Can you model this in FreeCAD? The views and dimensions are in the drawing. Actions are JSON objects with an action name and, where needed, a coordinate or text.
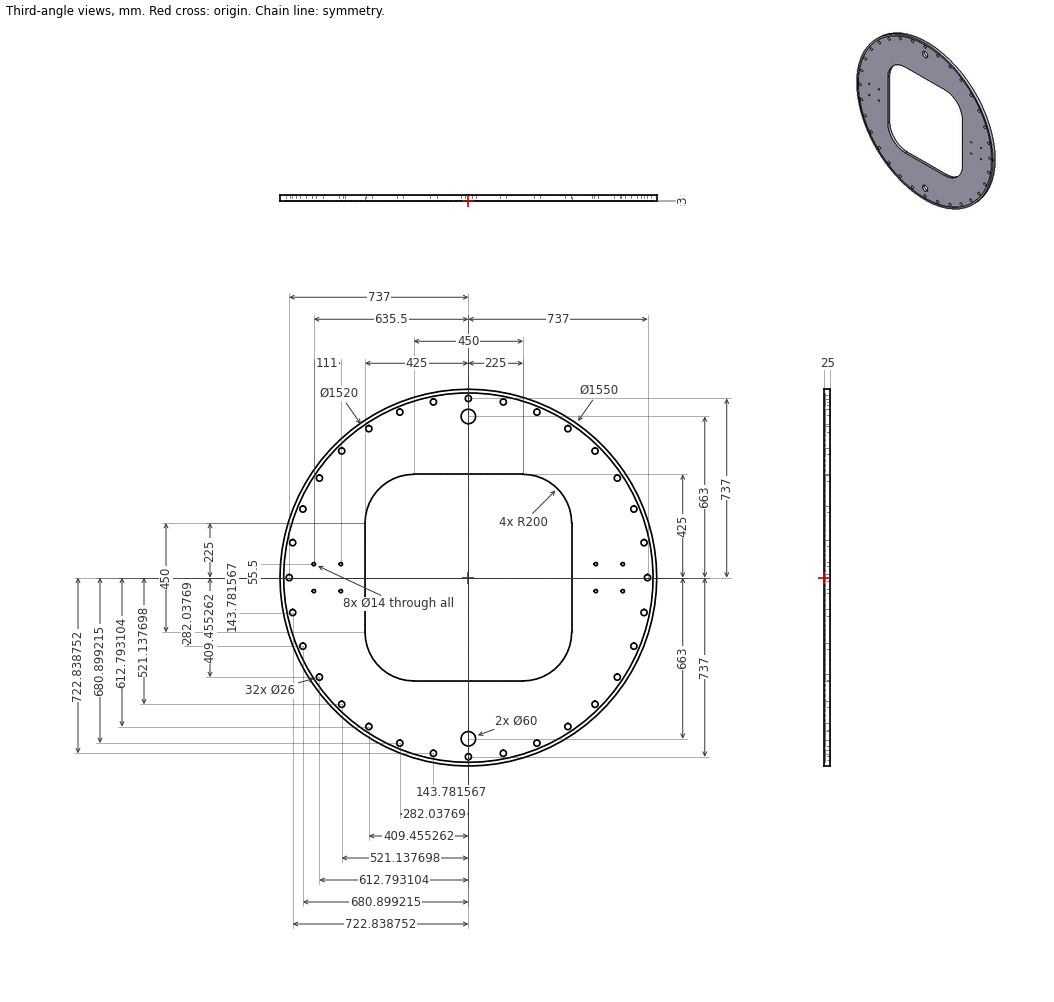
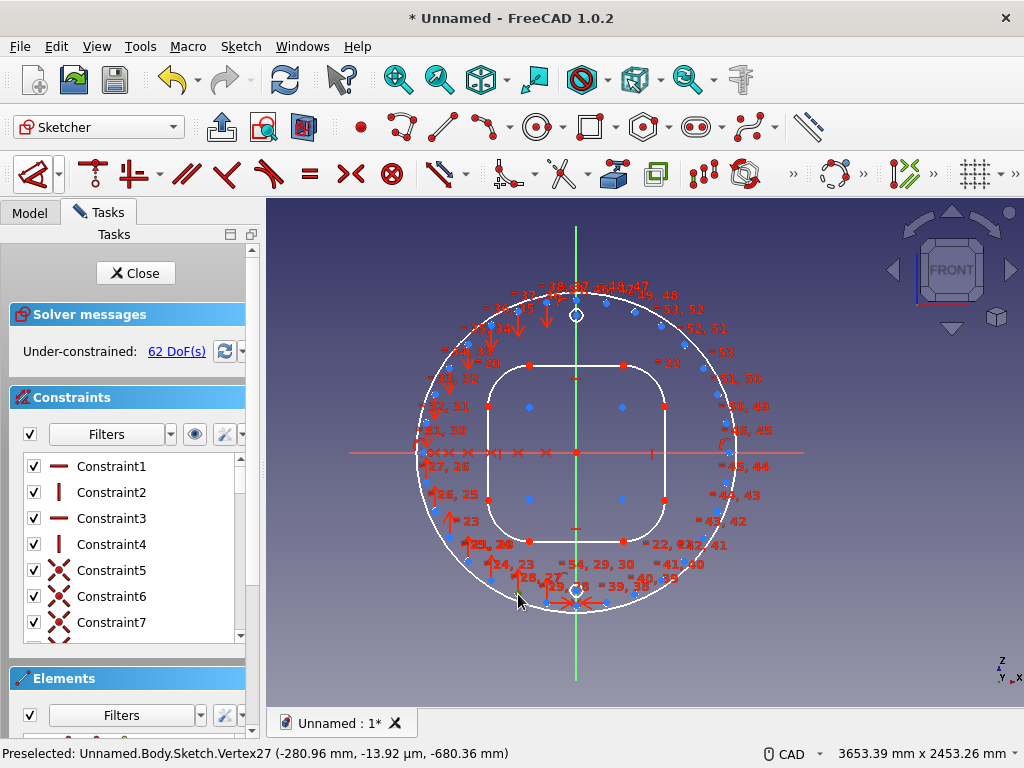
{"action": "left_click", "coordinate": [635, 595]}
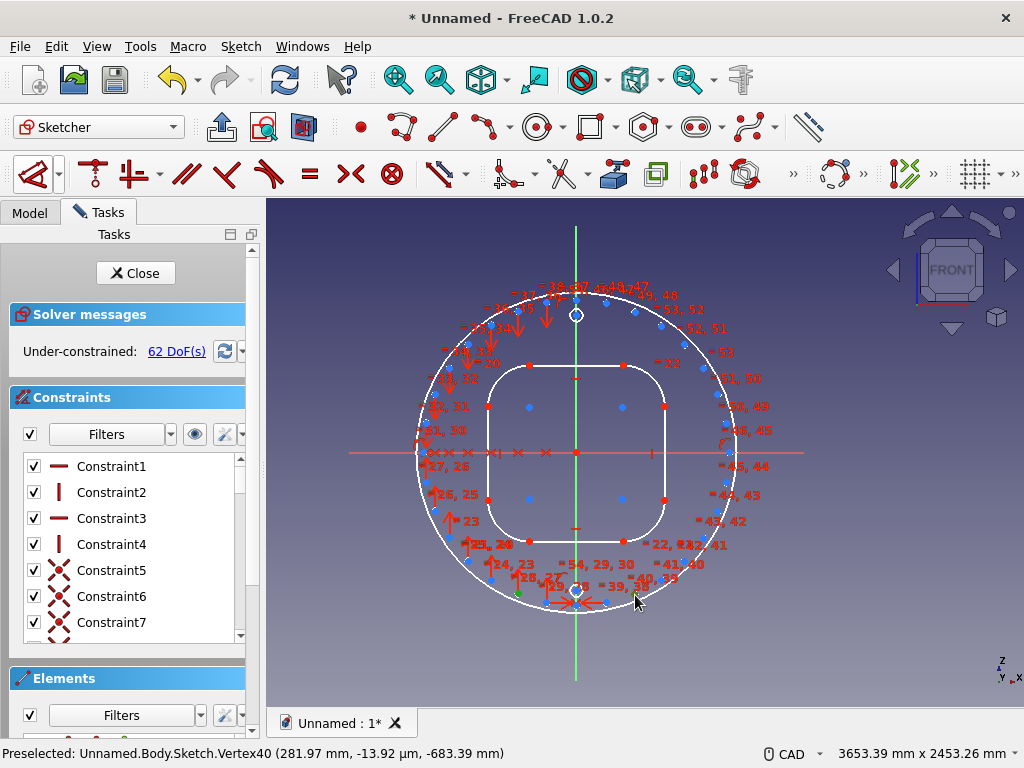
{"action": "left_click", "coordinate": [576, 647]}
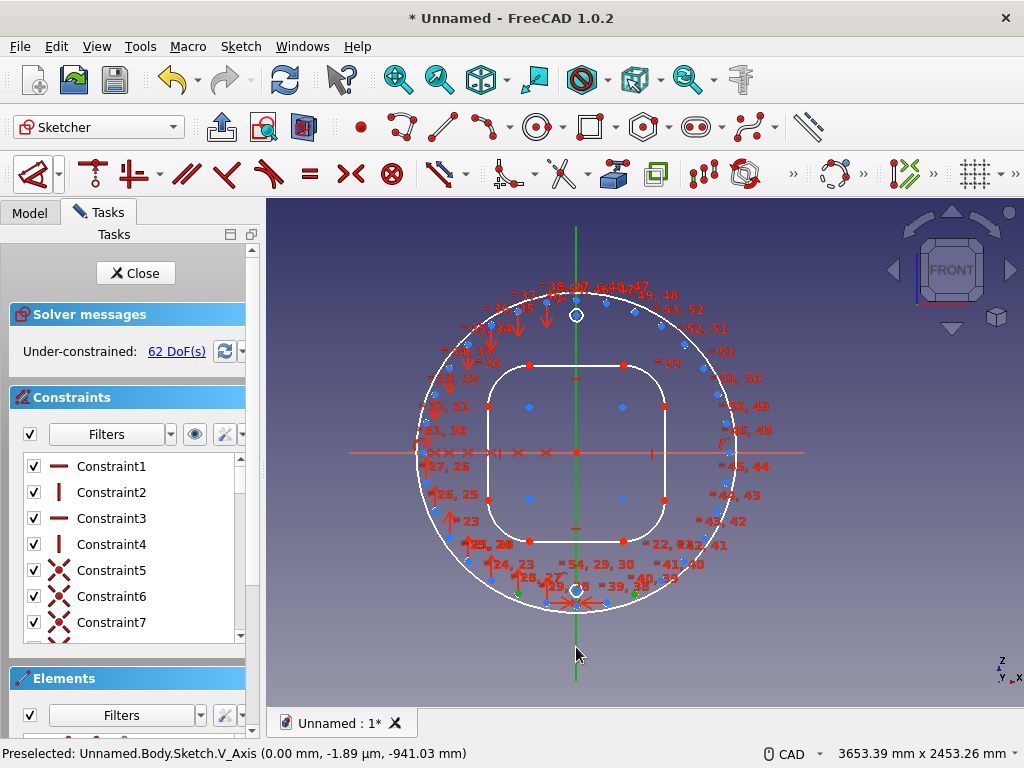
{"action": "left_click", "coordinate": [351, 174]}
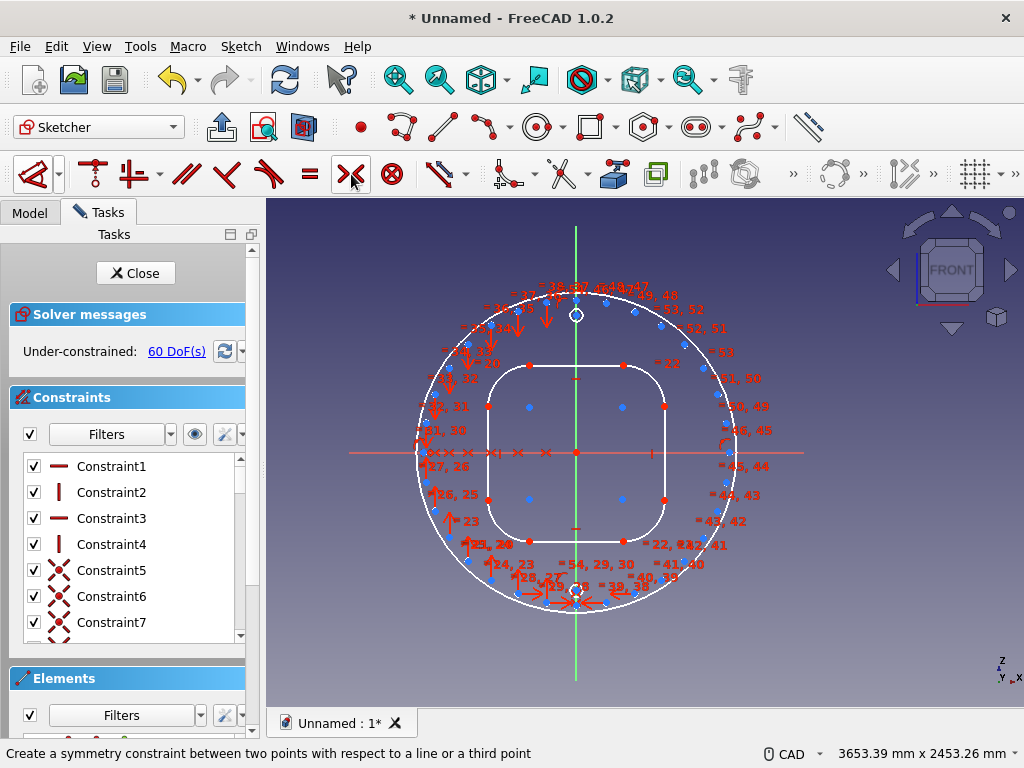
{"action": "left_click", "coordinate": [491, 580]}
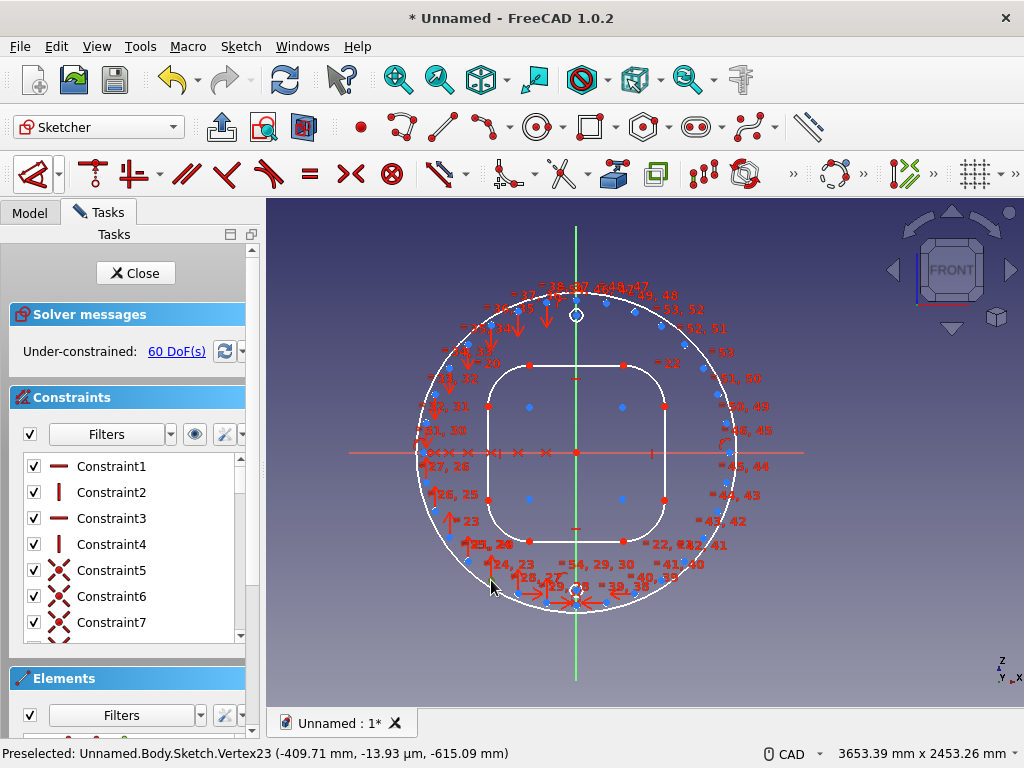
{"action": "left_click", "coordinate": [662, 580]}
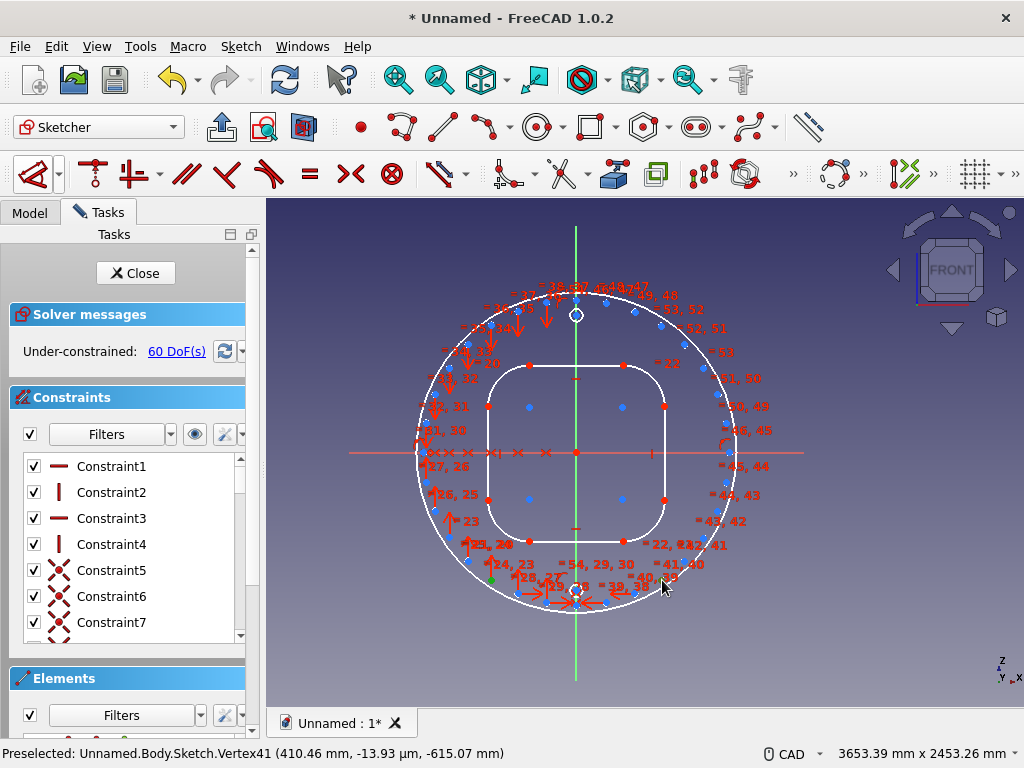
{"action": "left_click", "coordinate": [576, 647]}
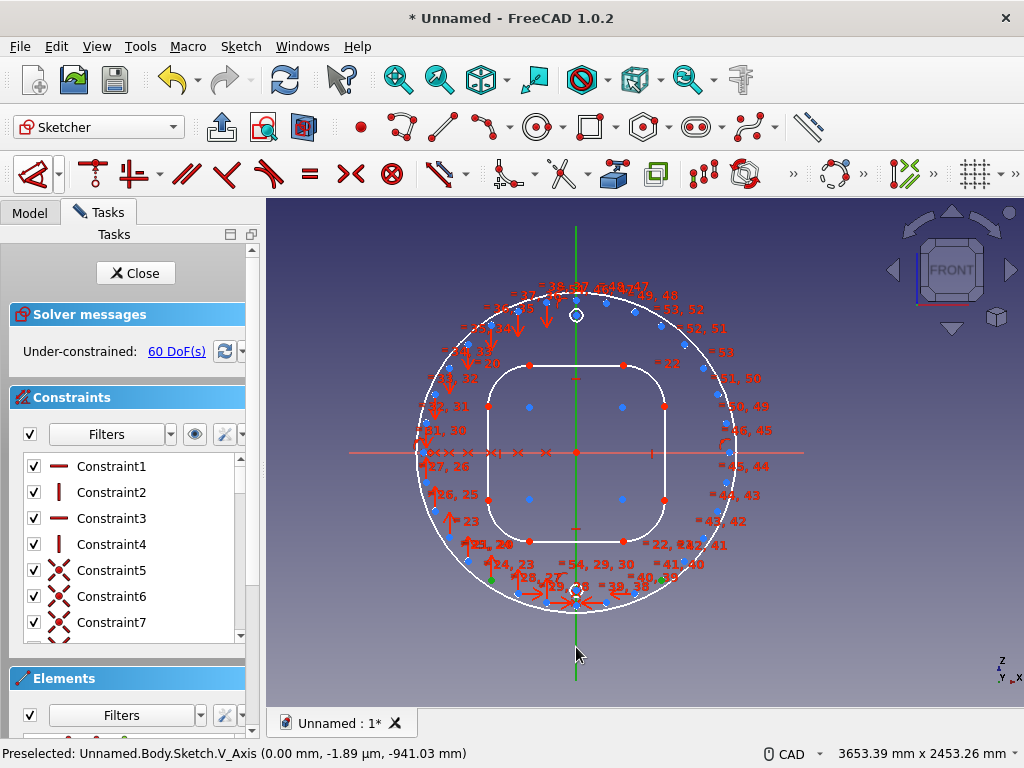
{"action": "left_click", "coordinate": [351, 174]}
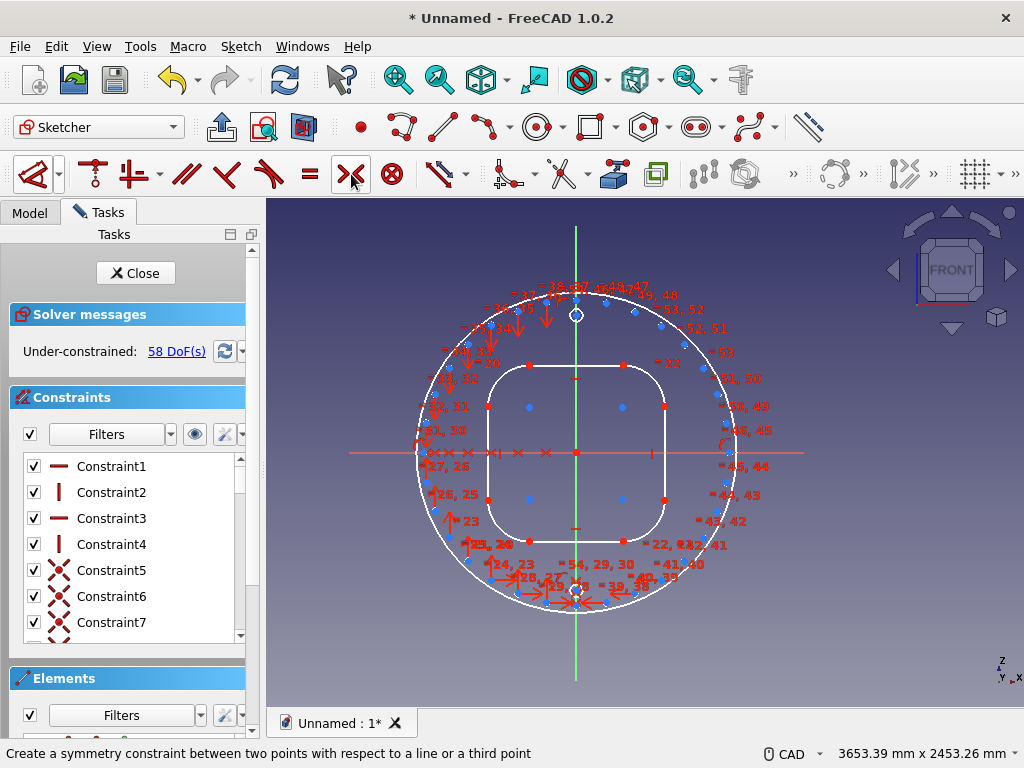
{"action": "left_click", "coordinate": [468, 561]}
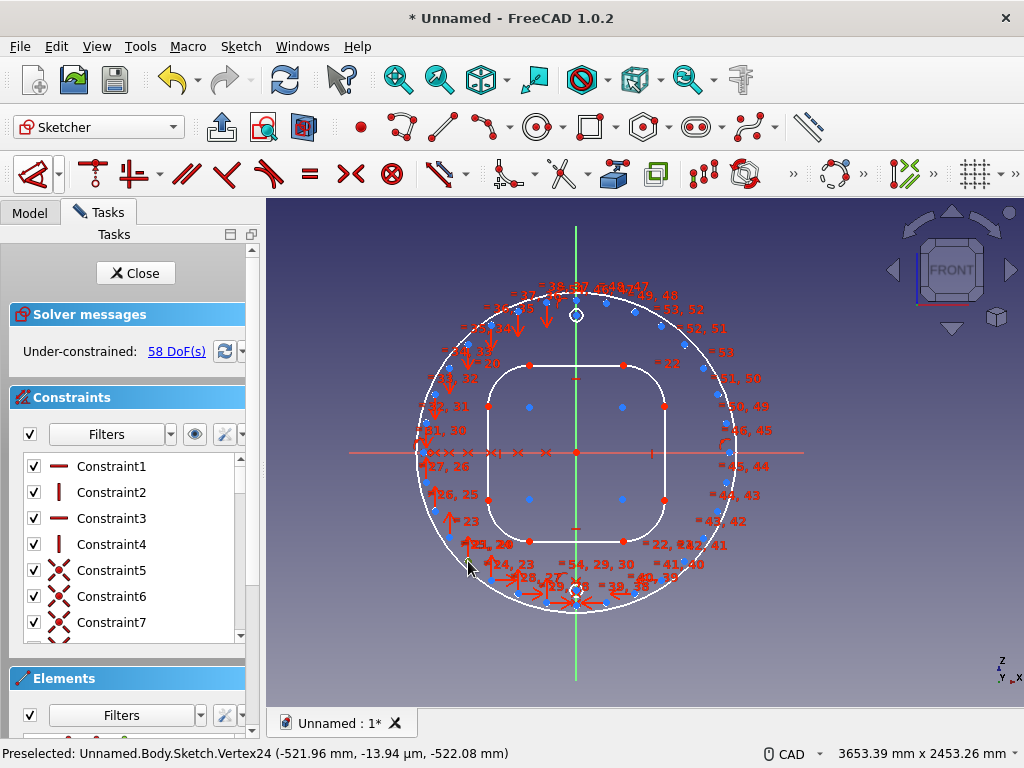
{"action": "left_click", "coordinate": [684, 561]}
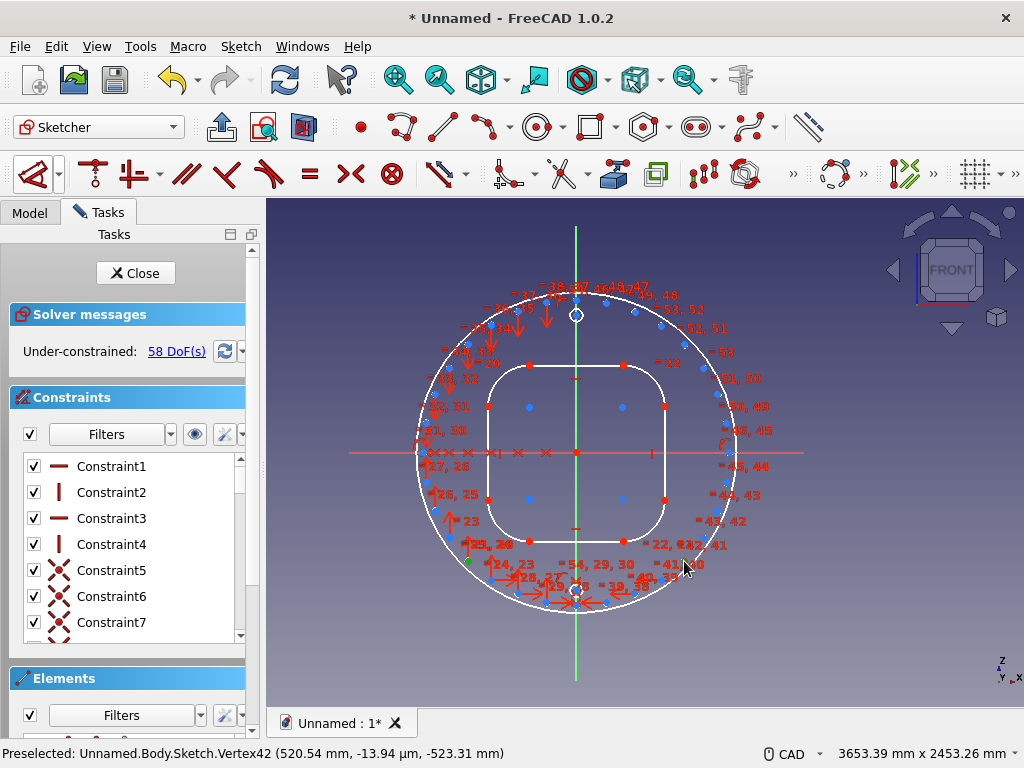
{"action": "left_click", "coordinate": [576, 647]}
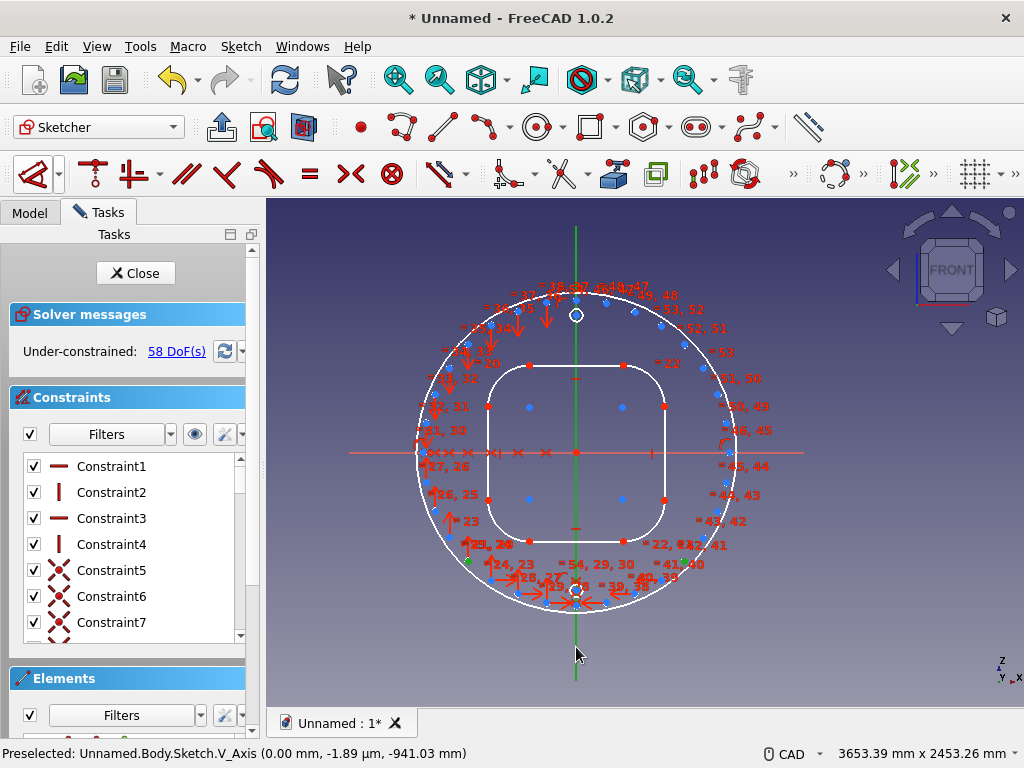
{"action": "left_click", "coordinate": [351, 174]}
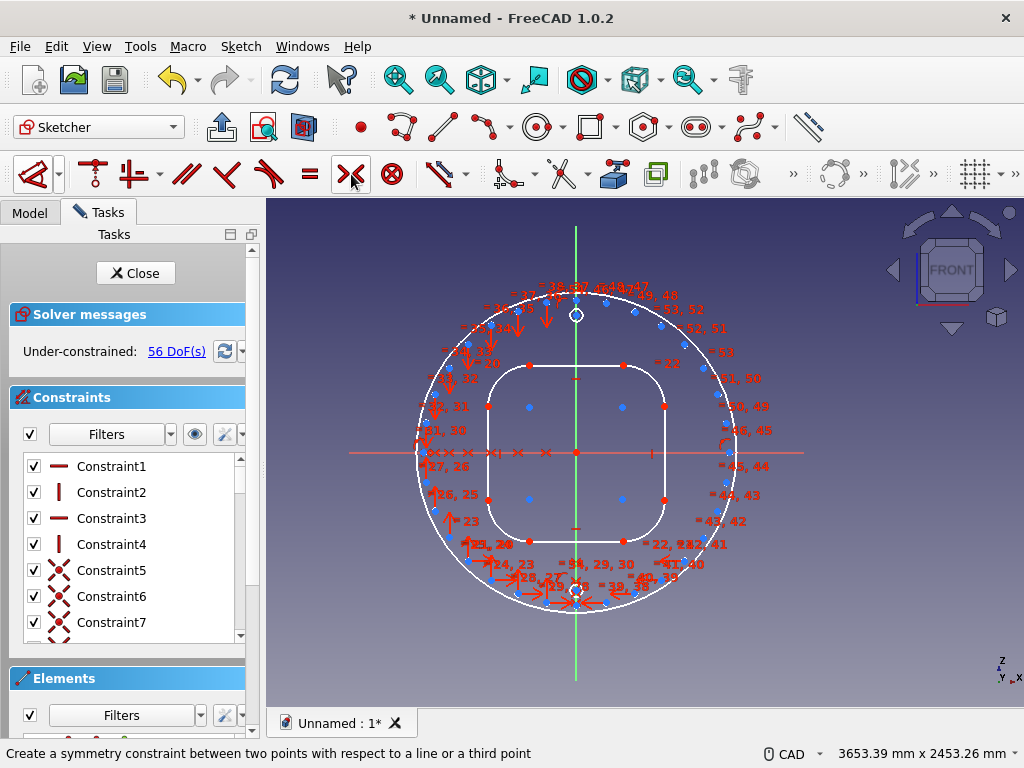
{"action": "left_click", "coordinate": [450, 537]}